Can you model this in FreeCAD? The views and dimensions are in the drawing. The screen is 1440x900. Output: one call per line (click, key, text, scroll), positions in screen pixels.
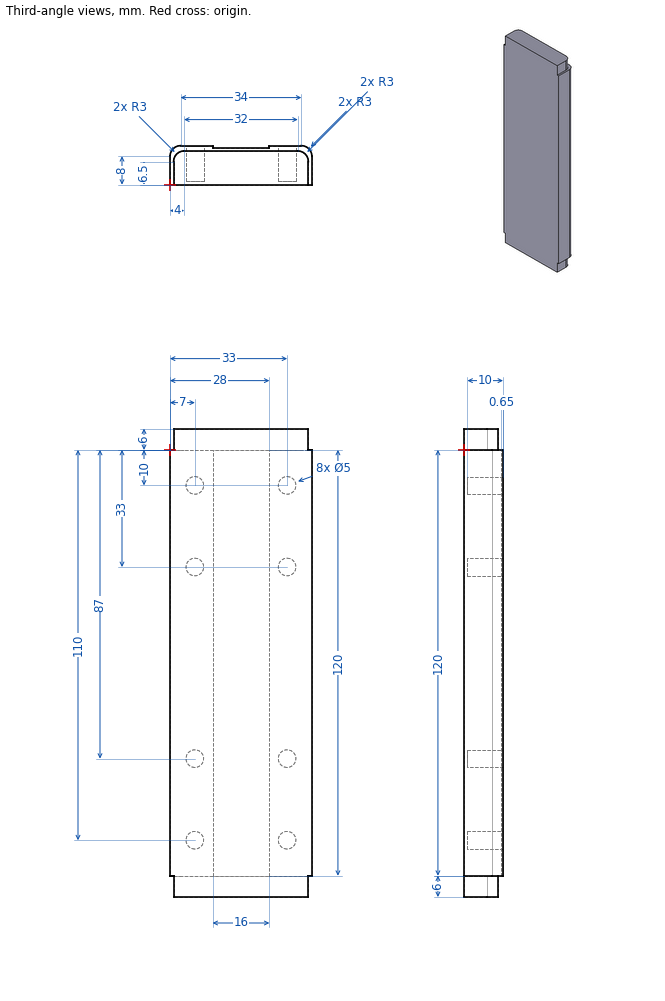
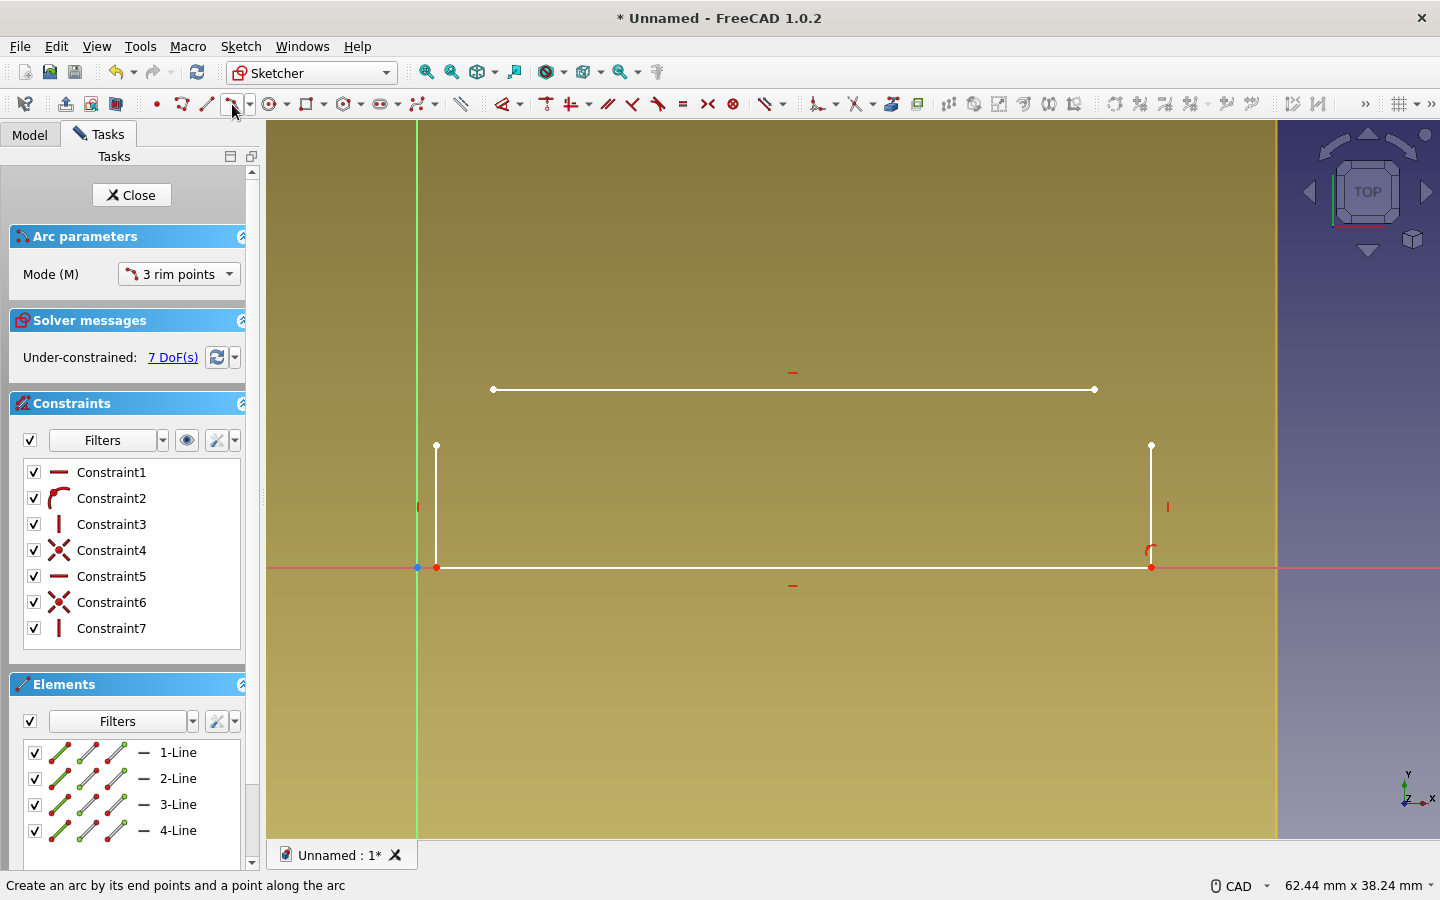
click(1094, 390)
click(1151, 446)
click(1134, 405)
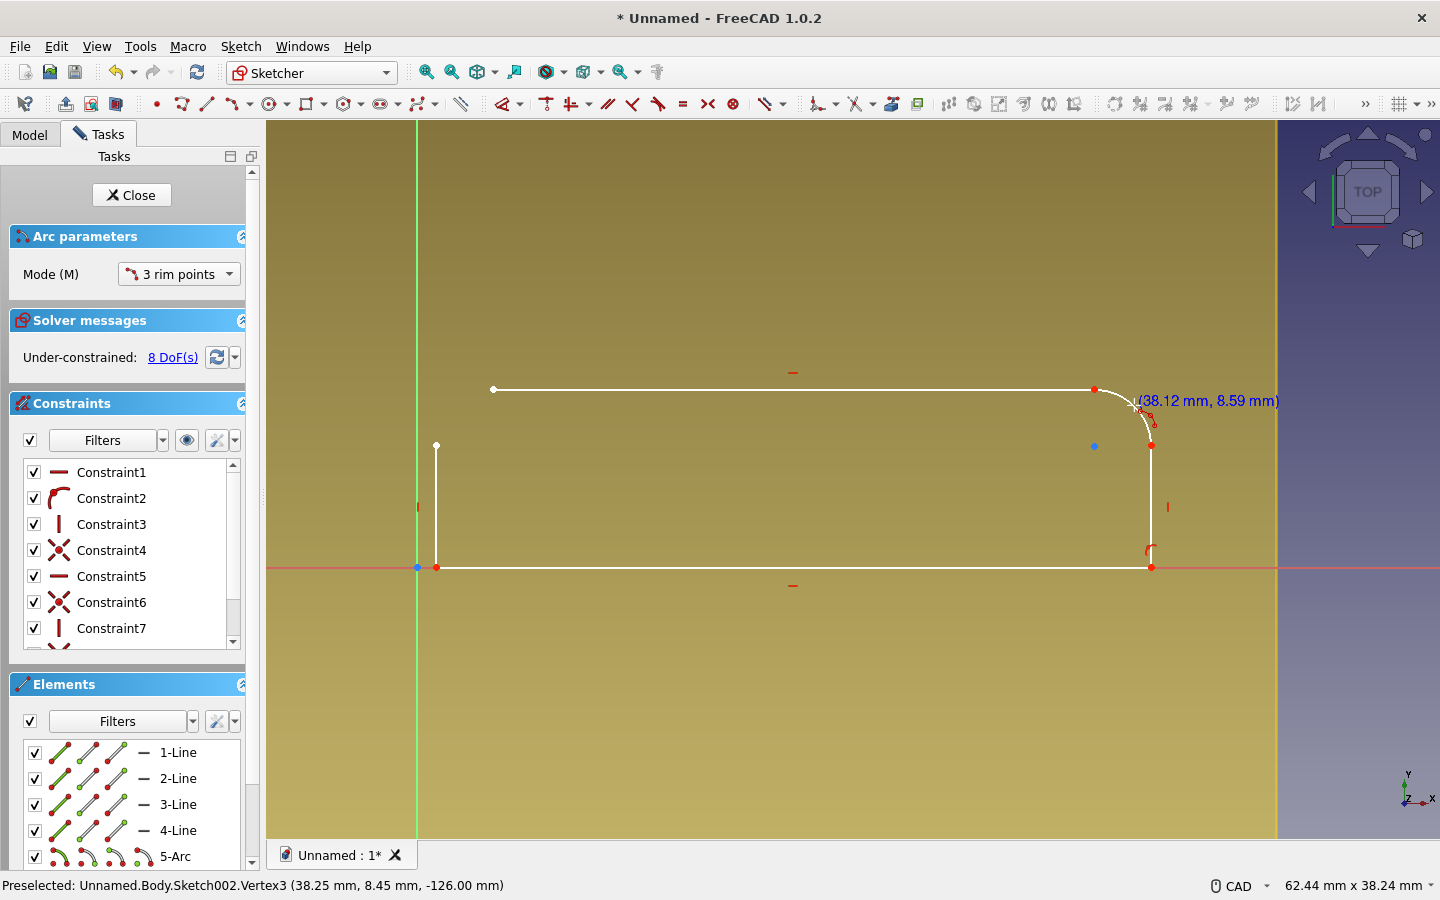
click(436, 446)
click(493, 390)
click(453, 405)
key(Escape)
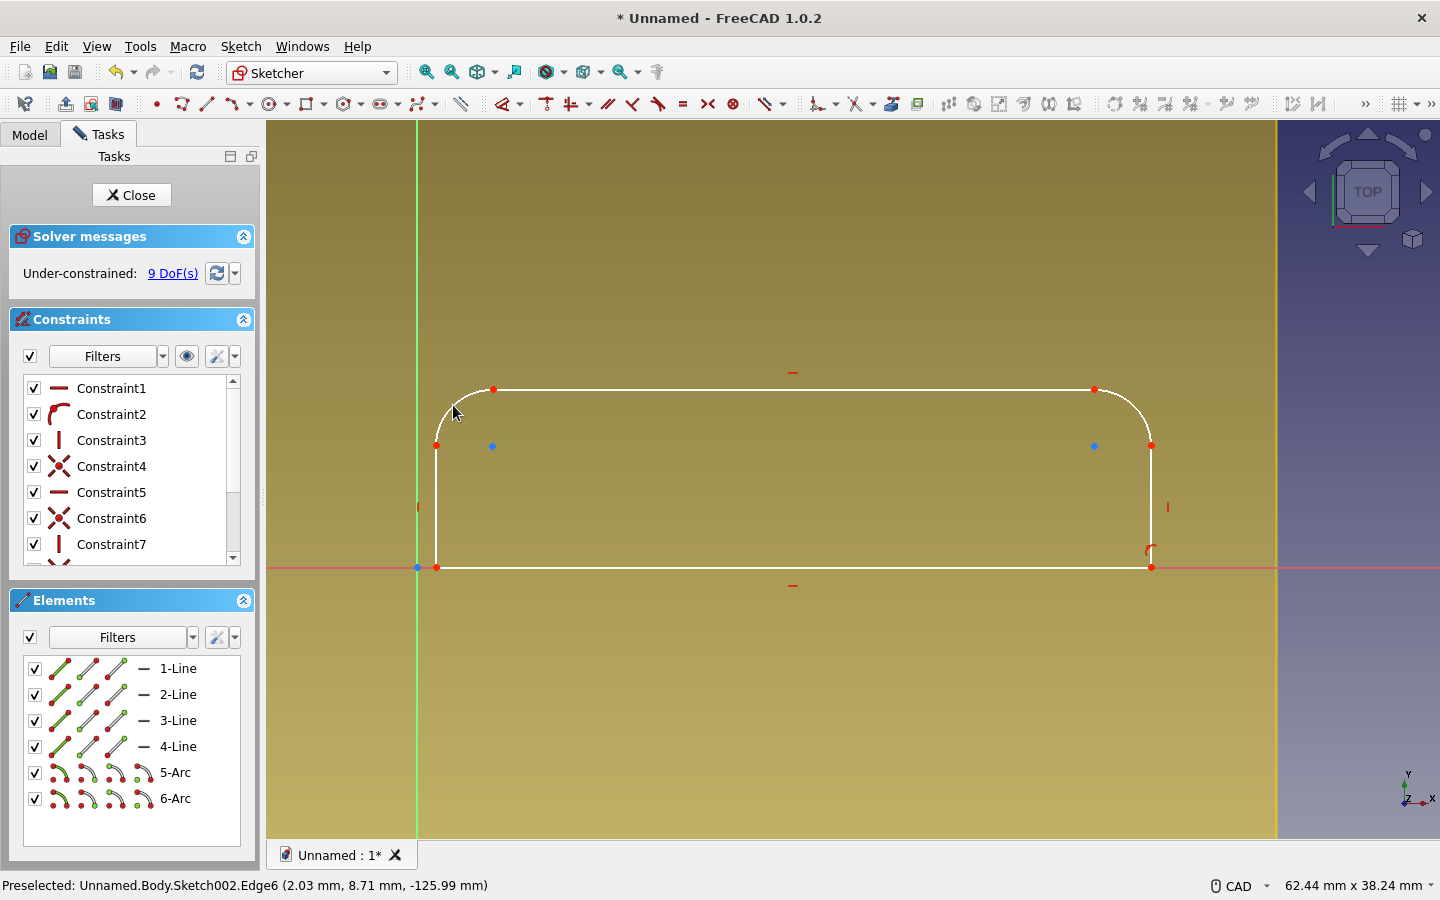
click(673, 390)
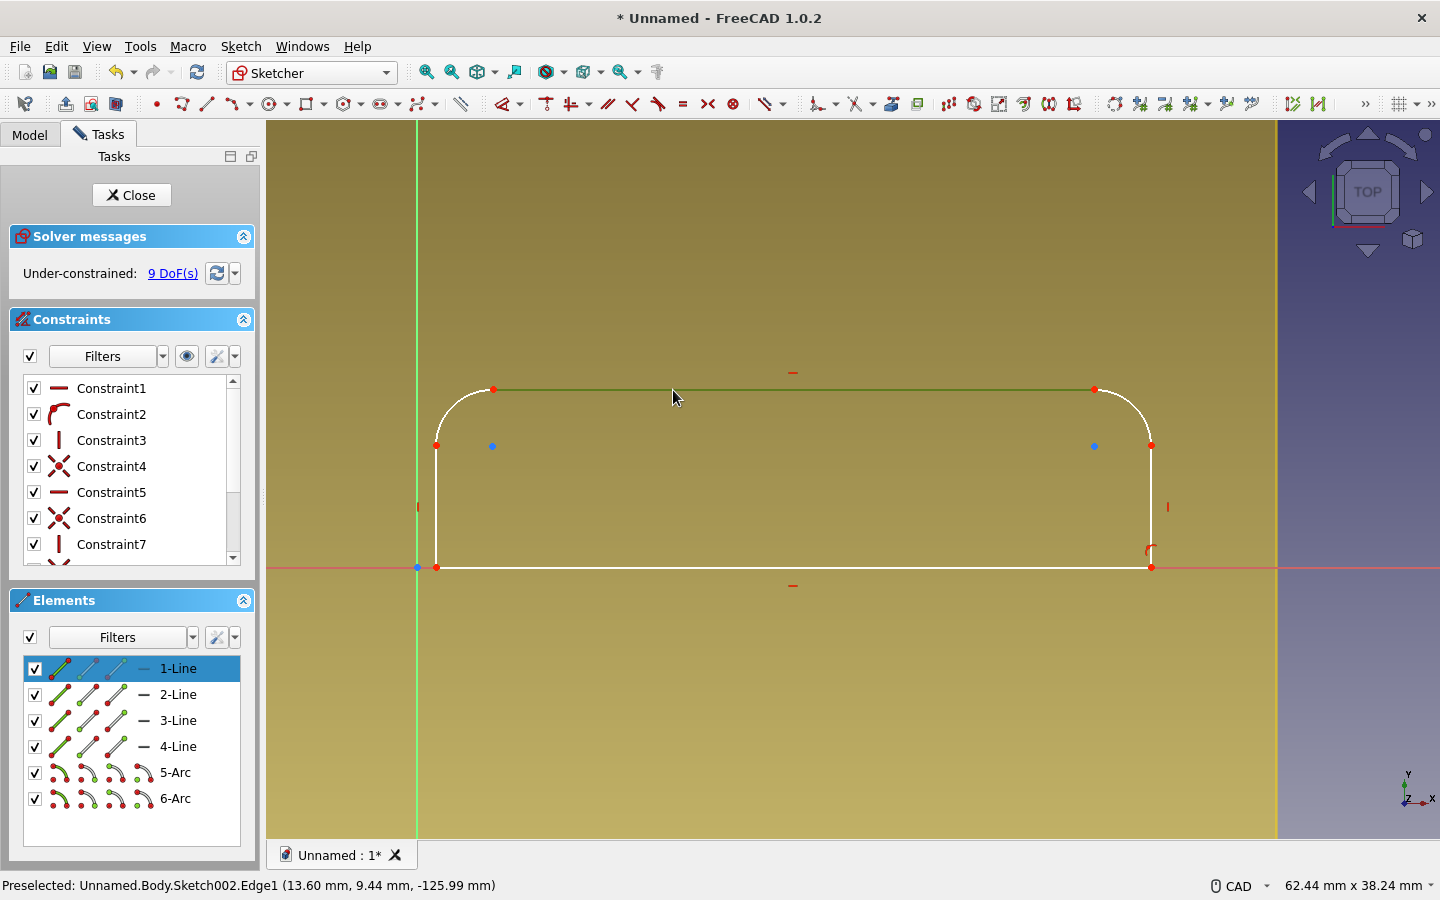
click(1145, 420)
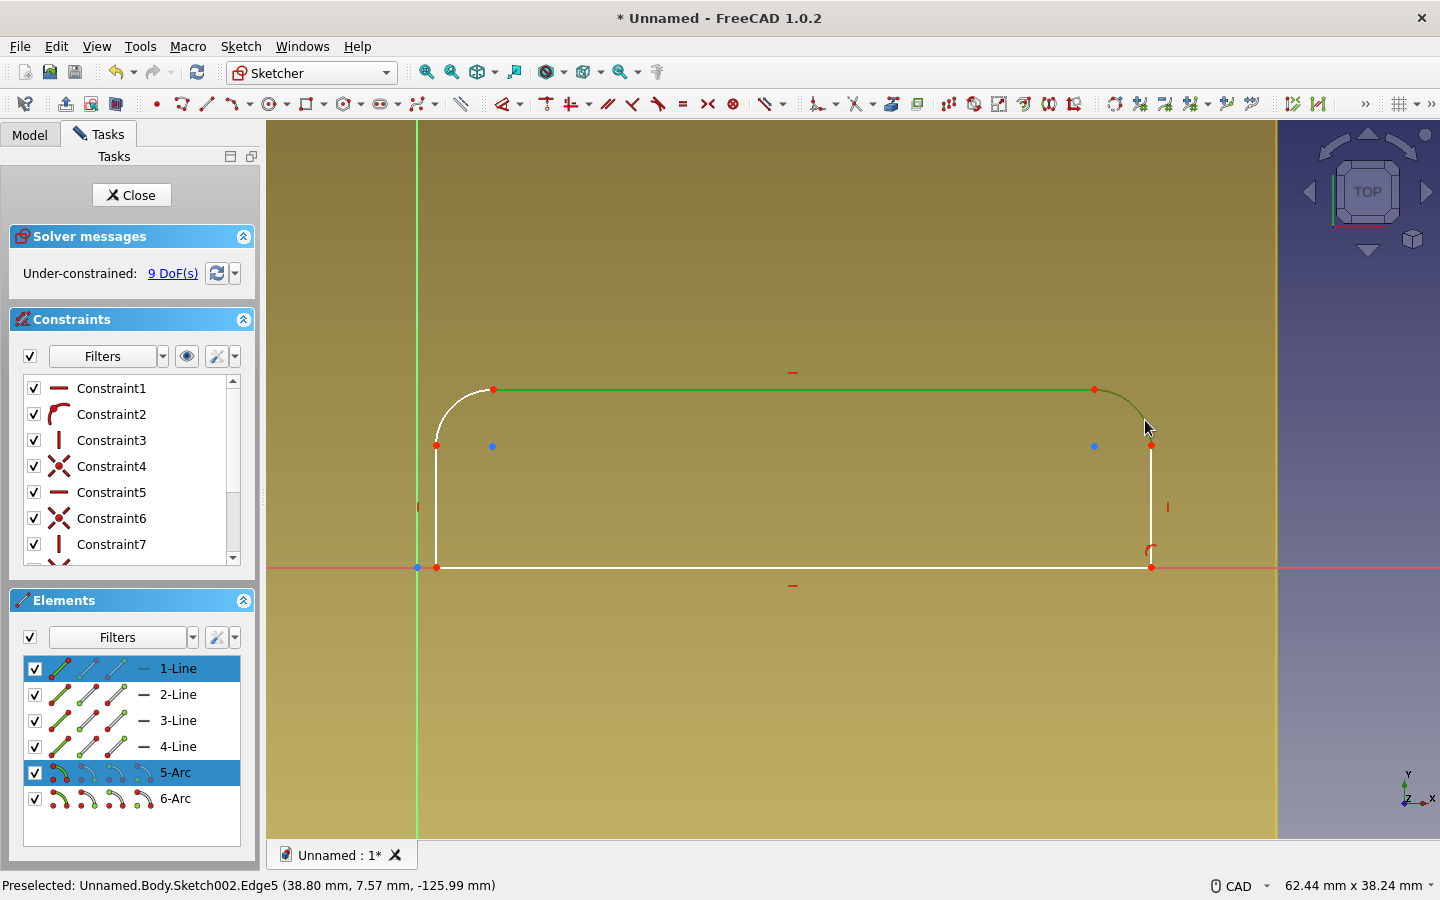
click(658, 104)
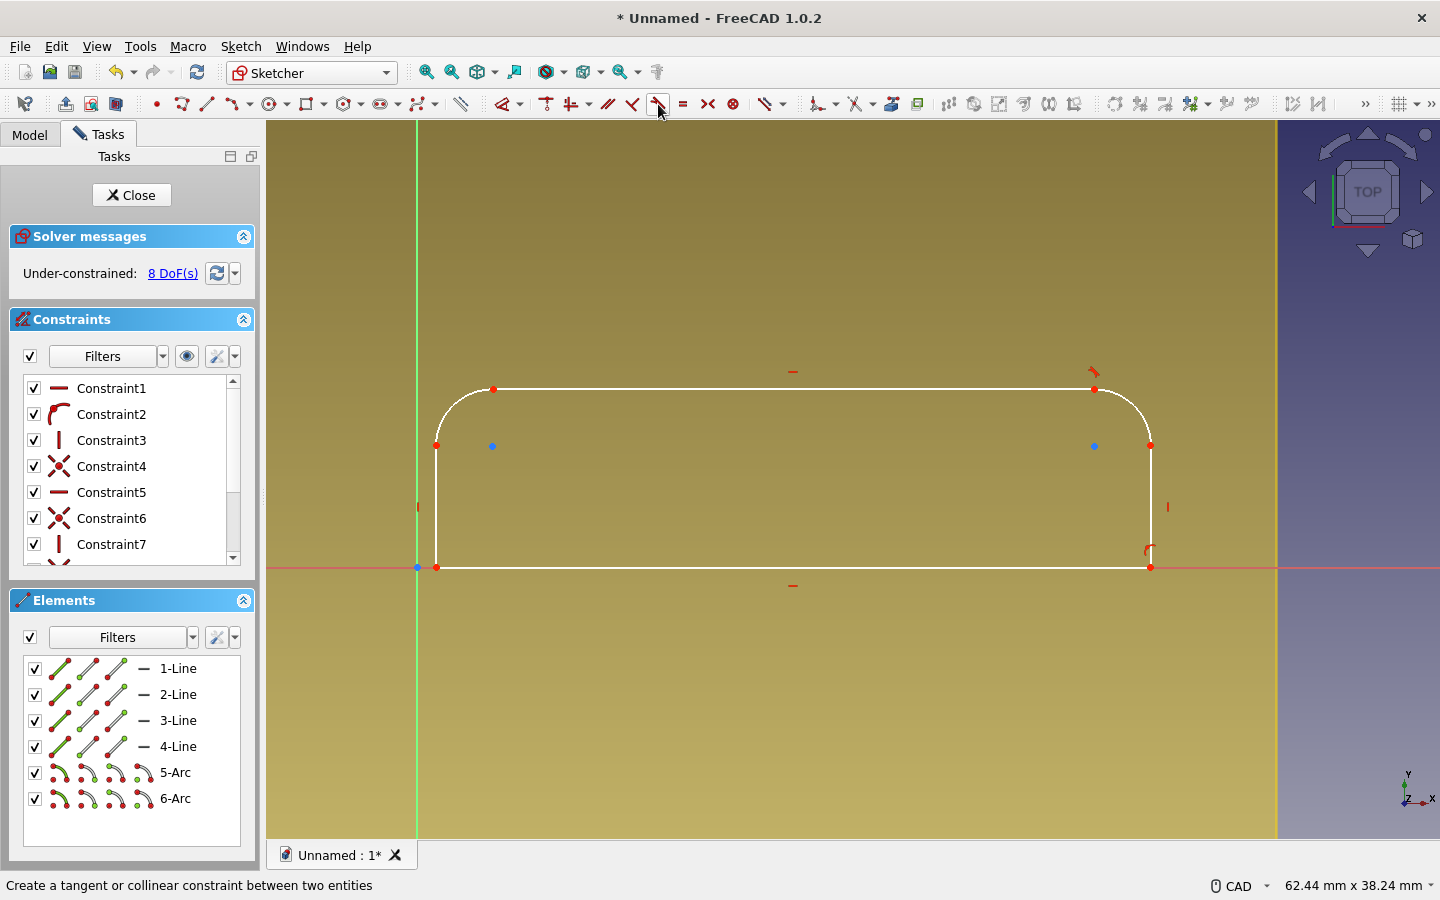
click(673, 389)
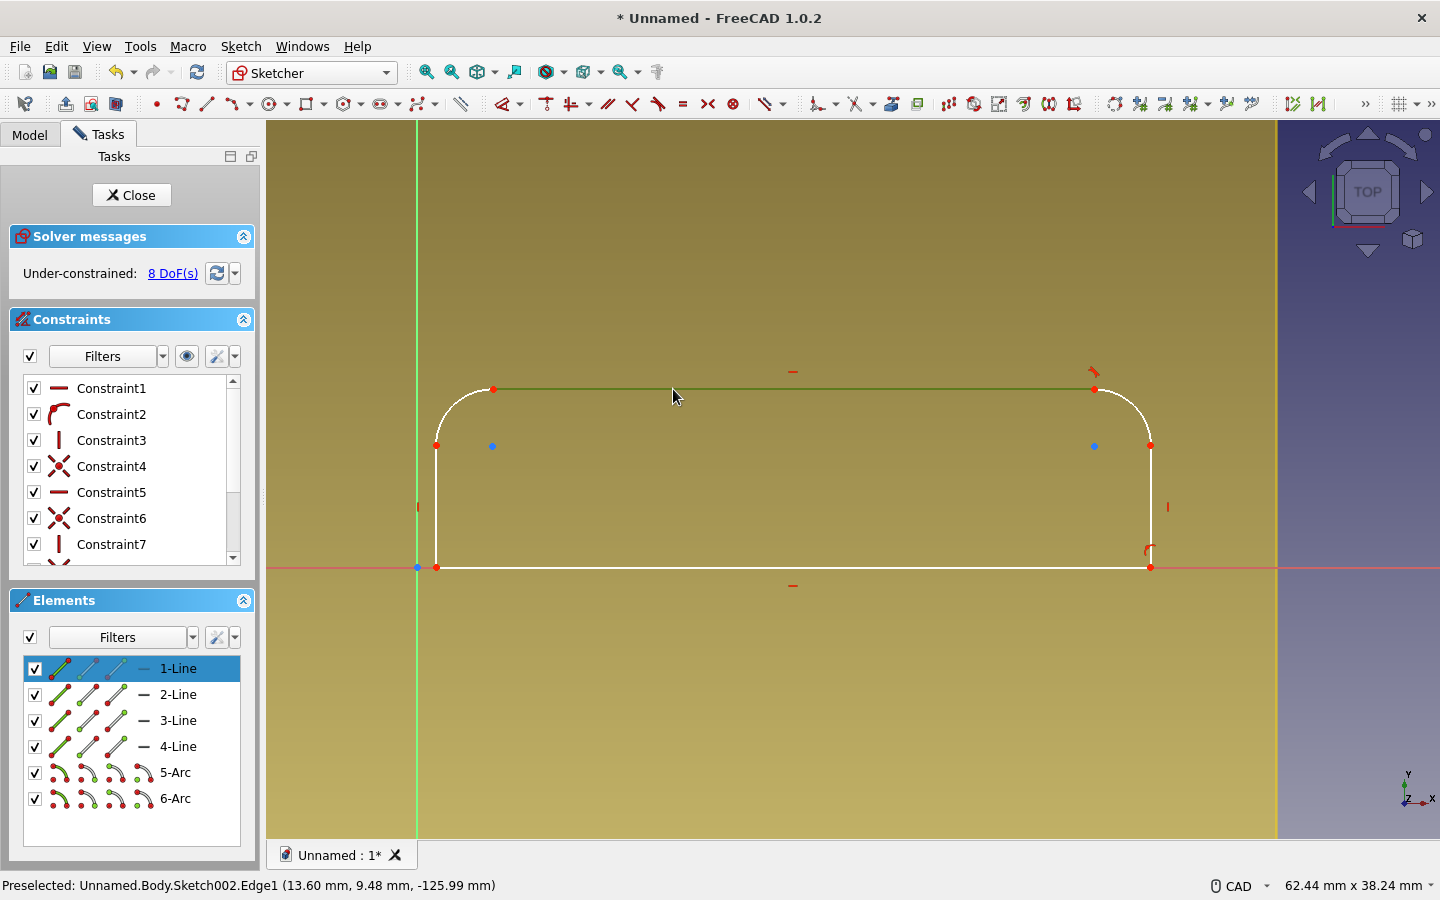
click(467, 395)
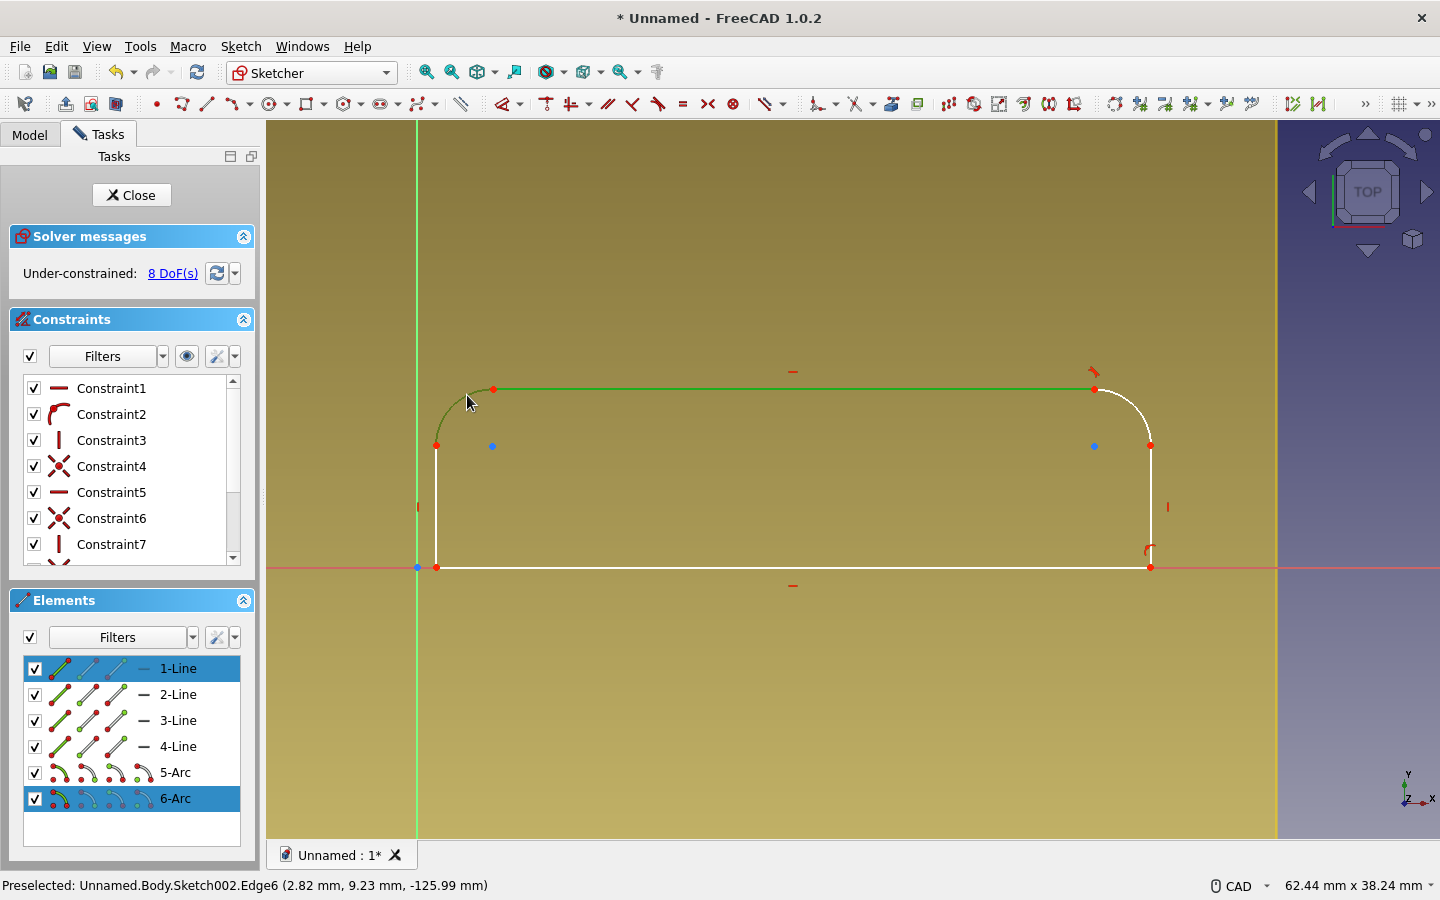
click(658, 104)